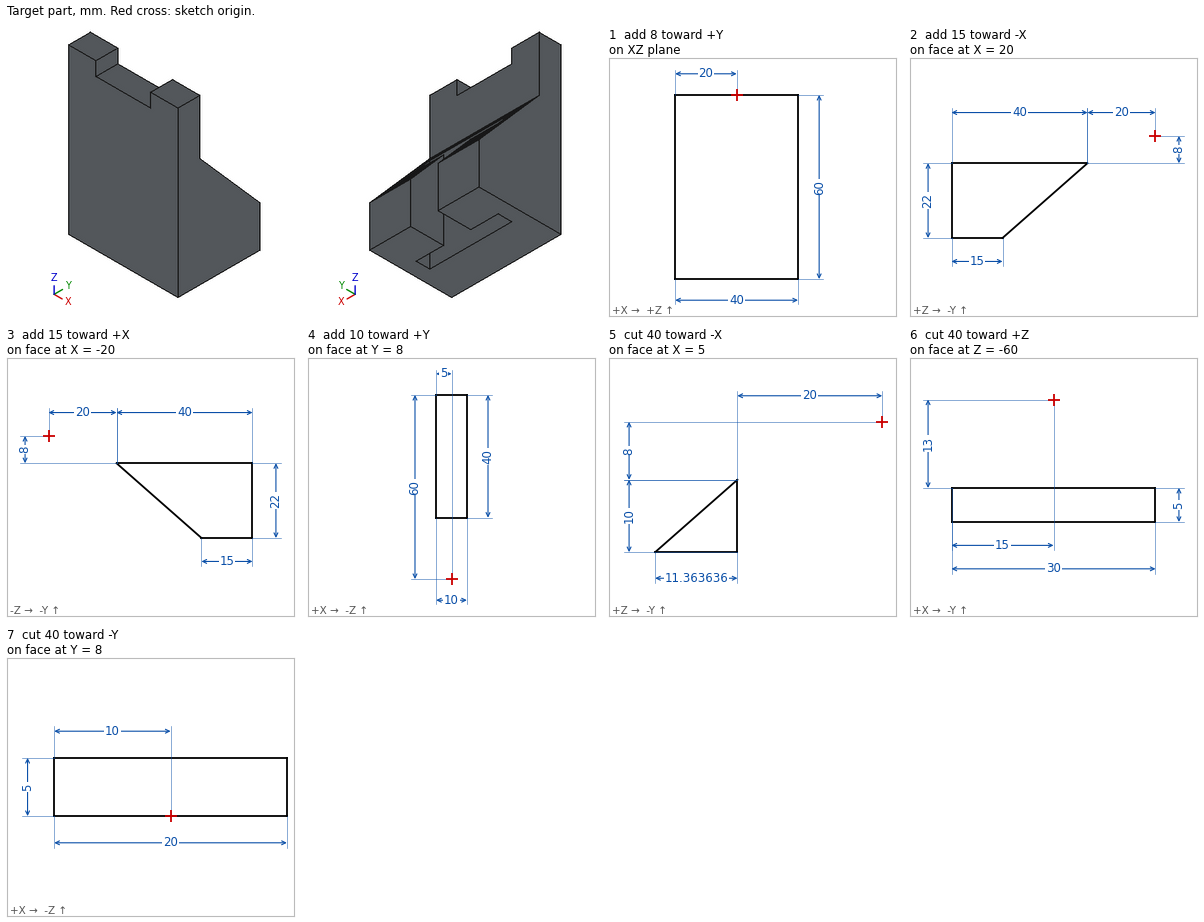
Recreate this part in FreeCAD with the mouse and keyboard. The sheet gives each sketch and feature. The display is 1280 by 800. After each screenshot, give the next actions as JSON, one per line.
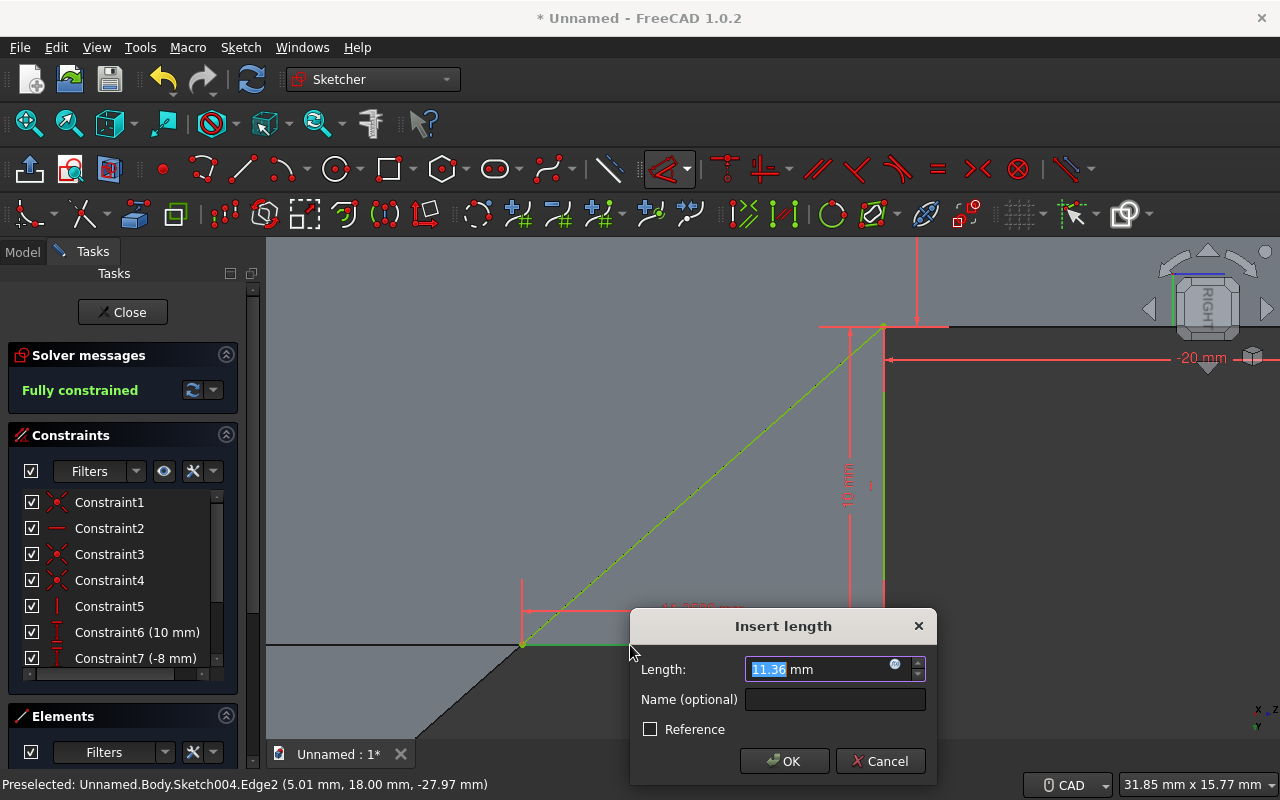
{"action": "type", "text": "11.363636"}
{"action": "key", "text": "Return"}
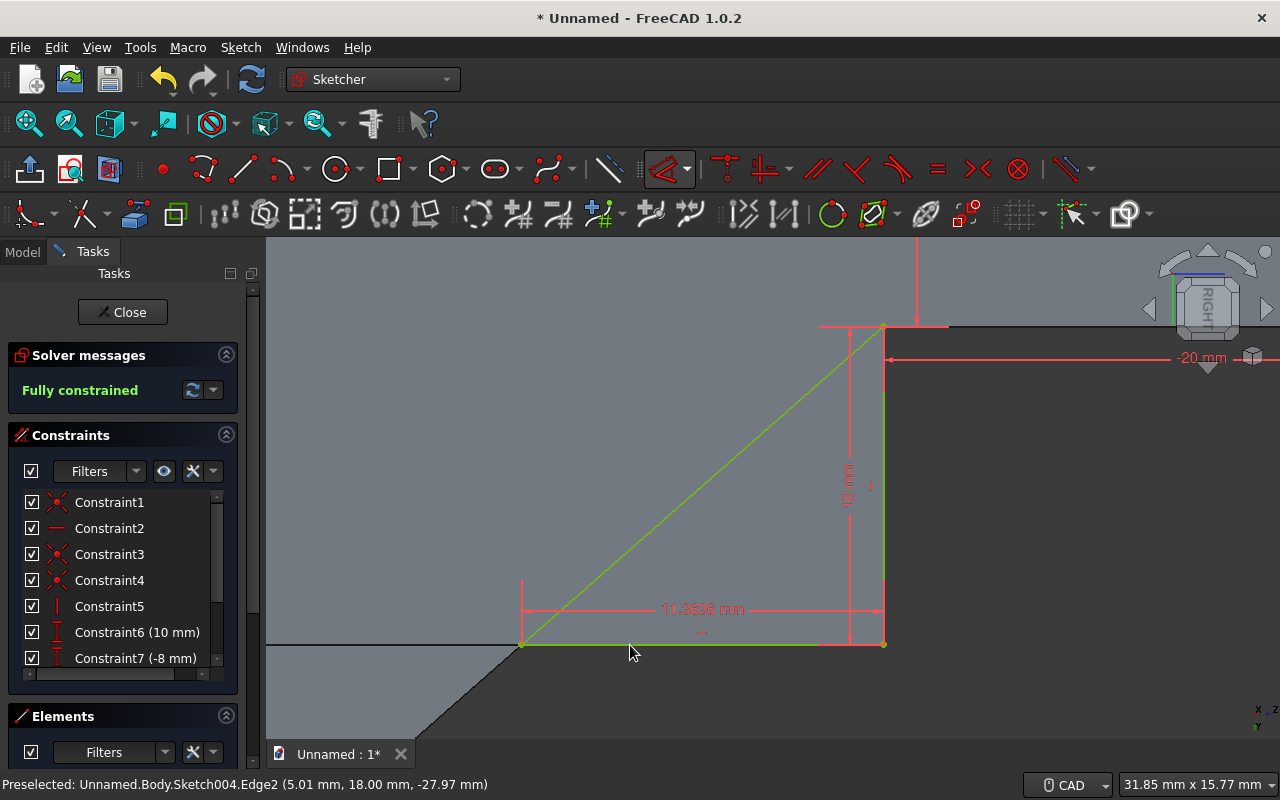
{"action": "left_click", "coordinate": [123, 312]}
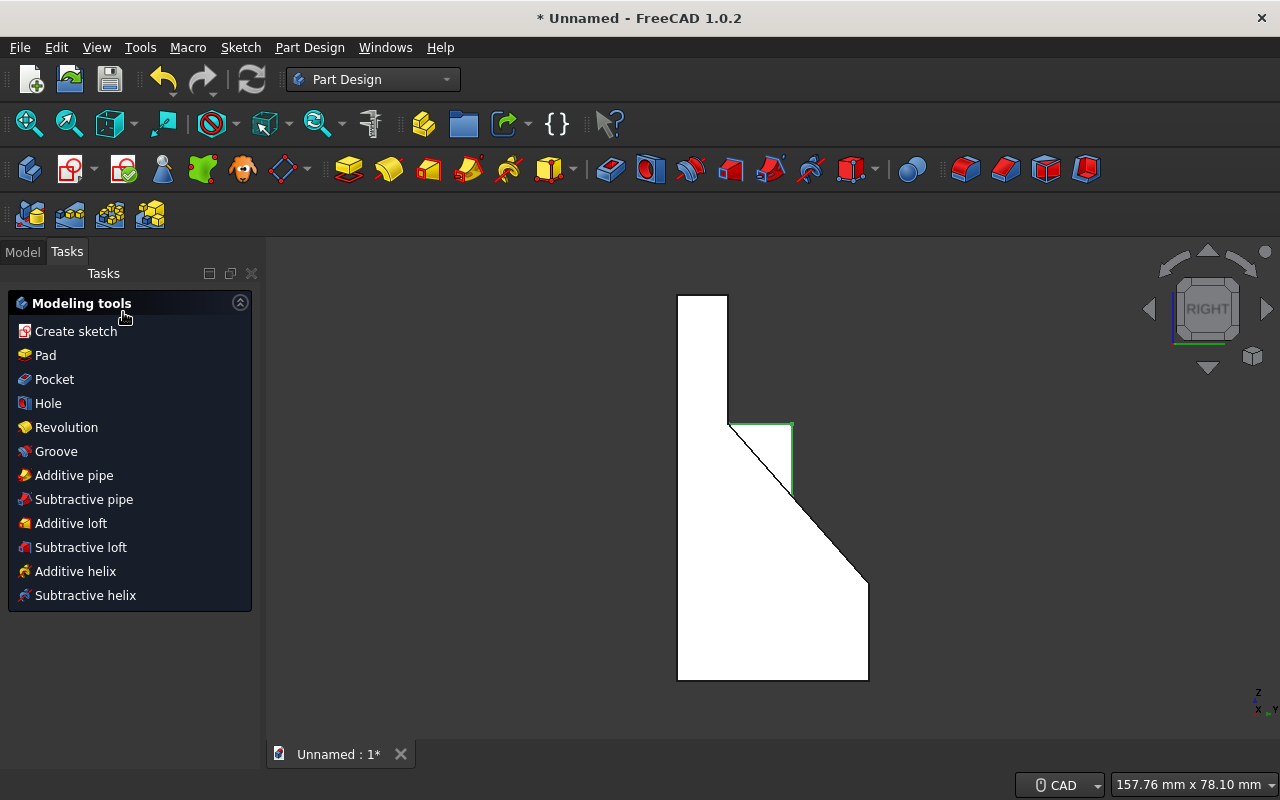
{"action": "left_click", "coordinate": [612, 170]}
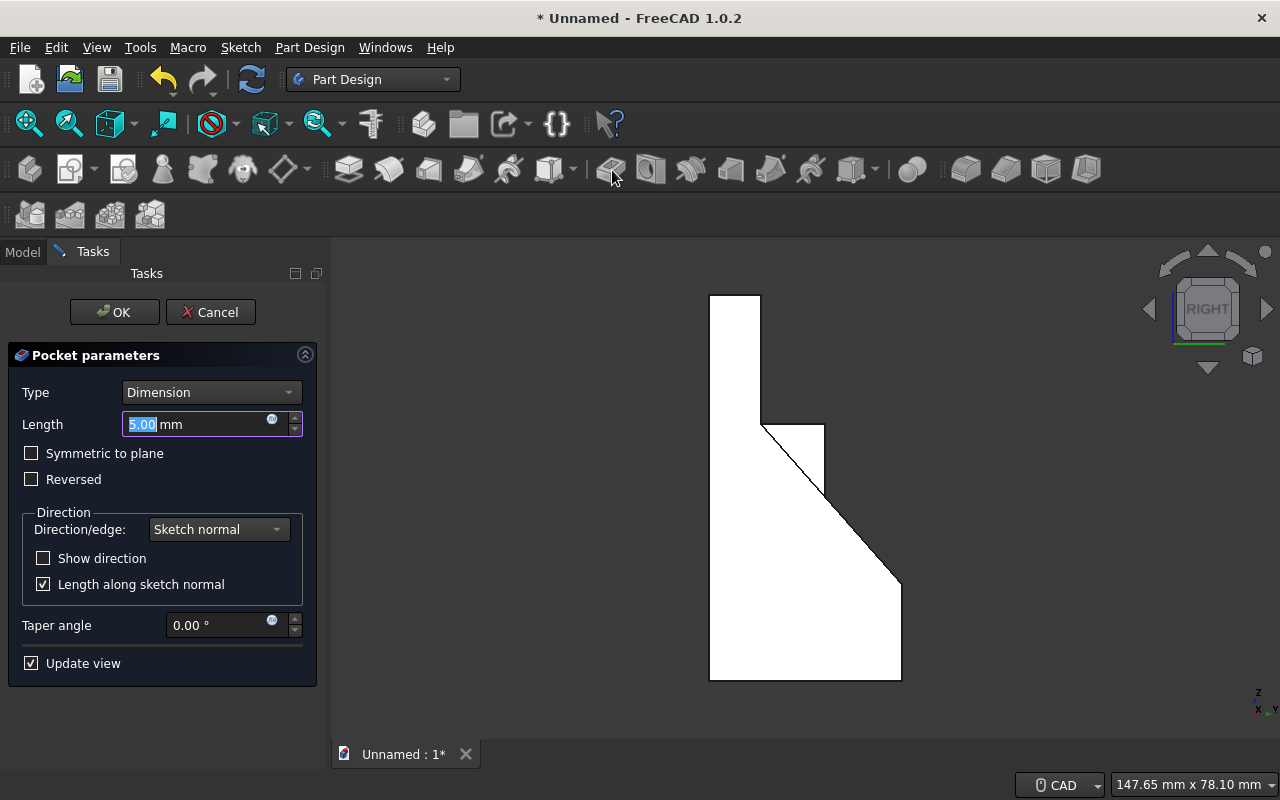
{"action": "type", "text": "40"}
{"action": "key", "text": "Tab"}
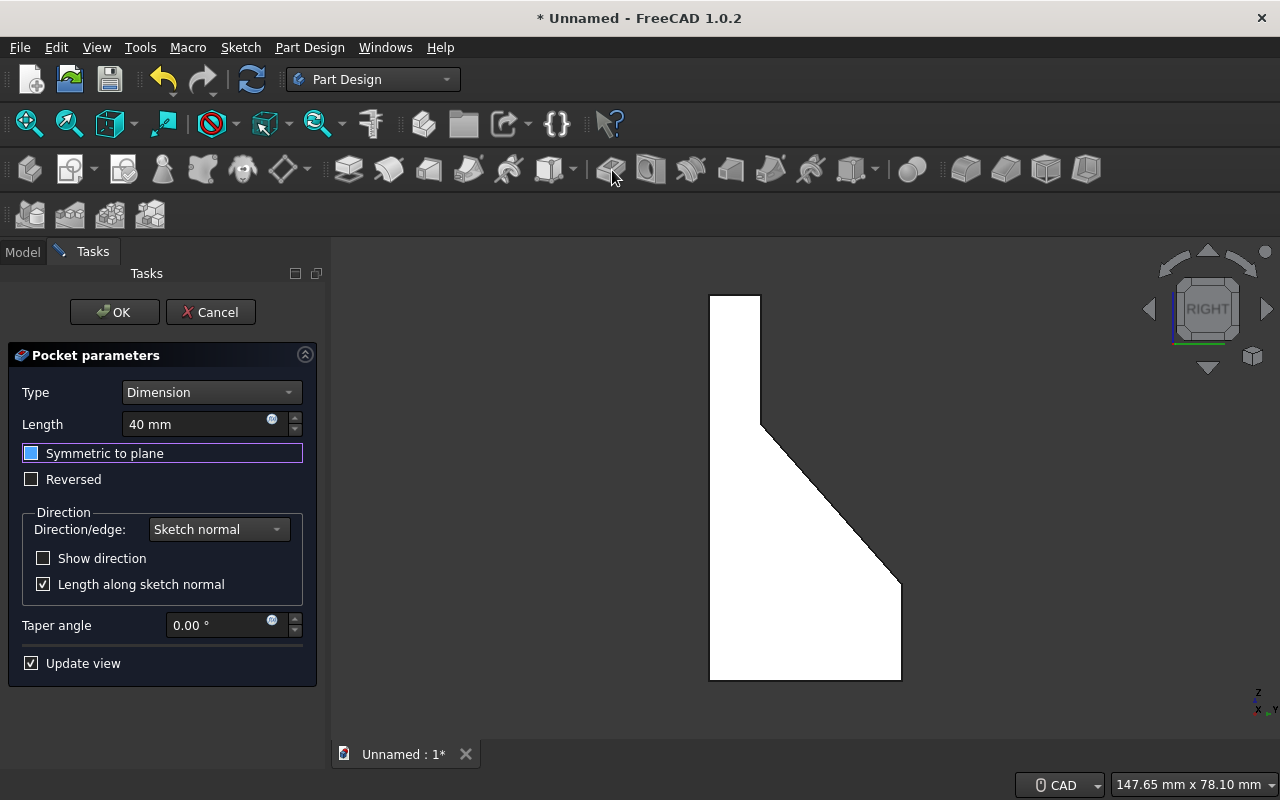
{"action": "left_click", "coordinate": [115, 312]}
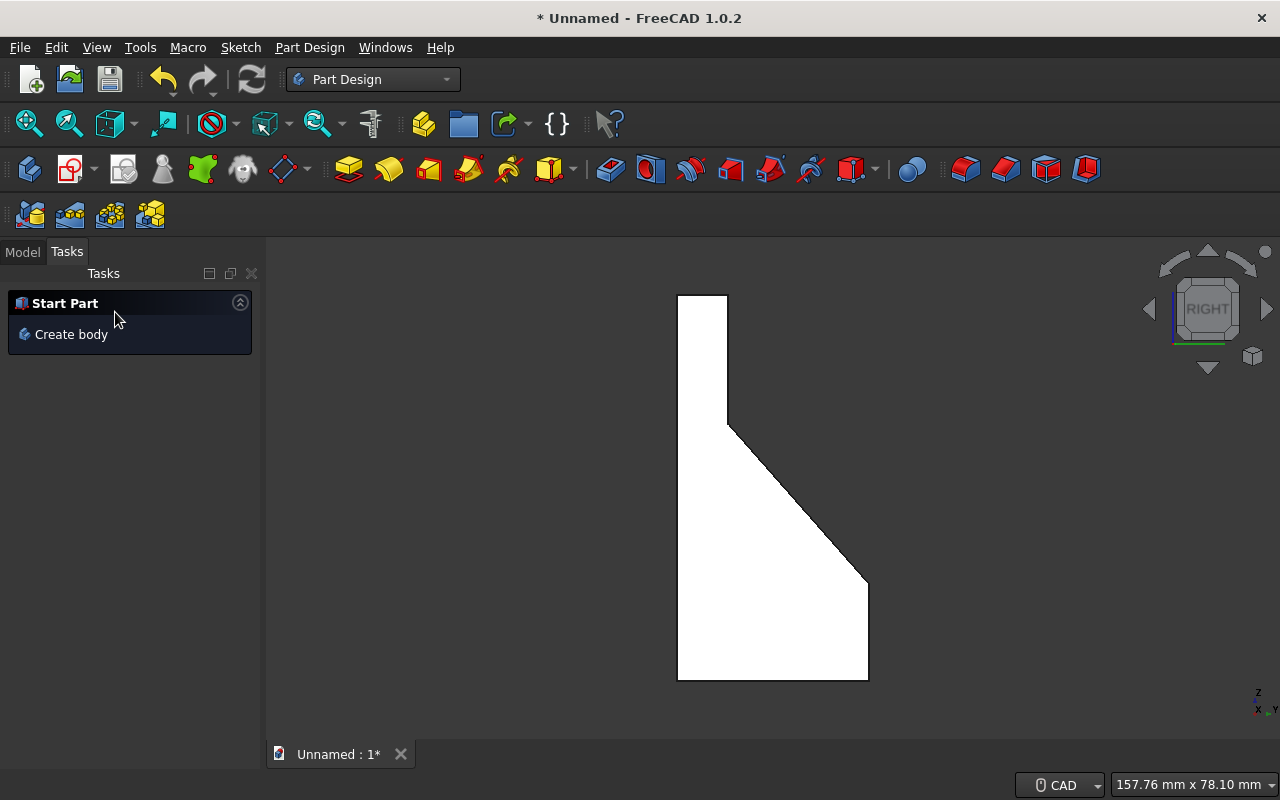
{"action": "key", "text": "5"}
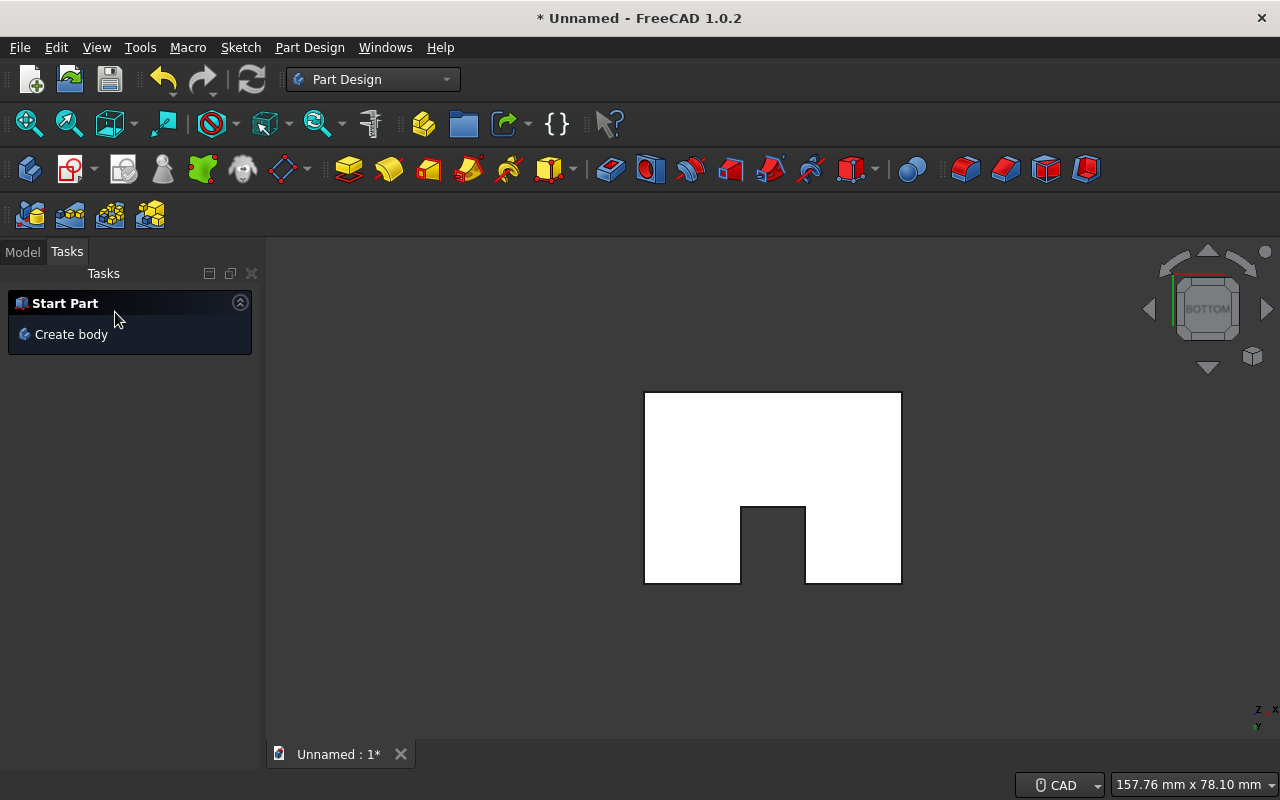
{"action": "left_click", "coordinate": [30, 124]}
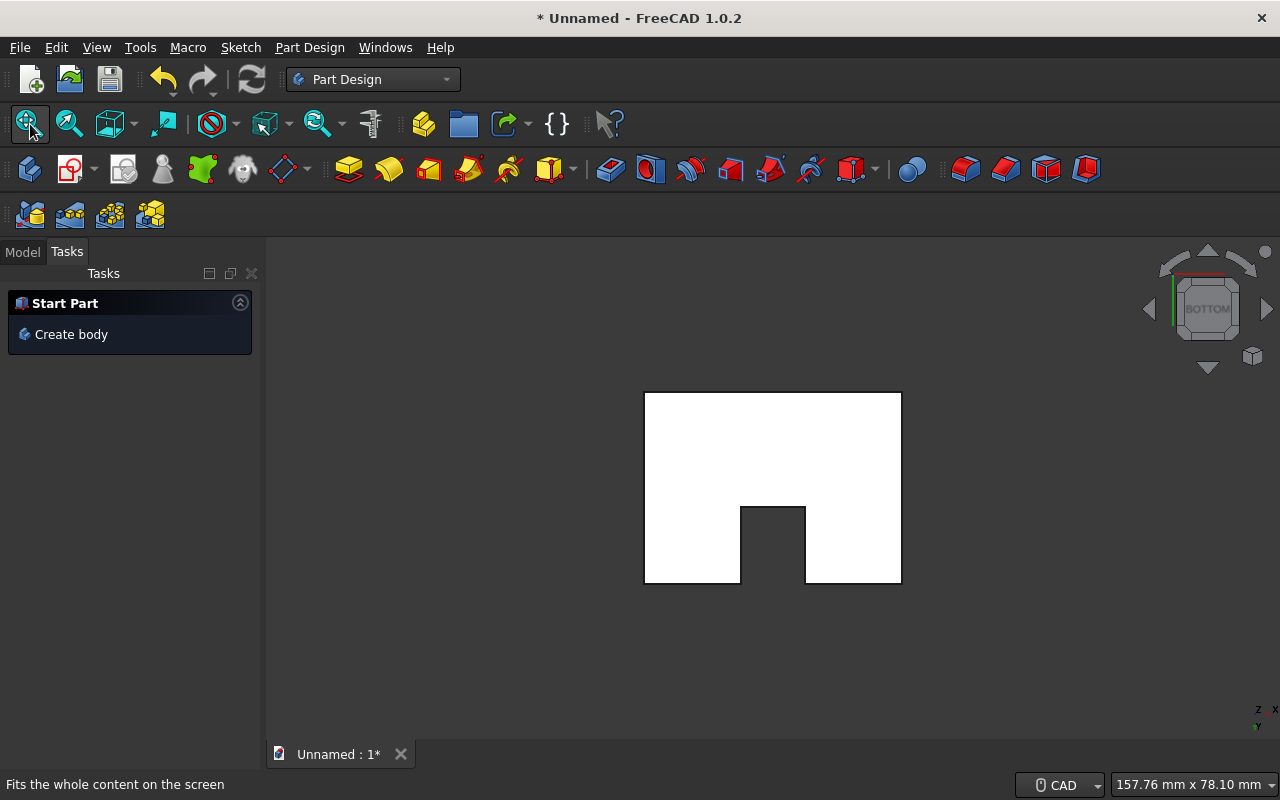
{"action": "left_click", "coordinate": [846, 459]}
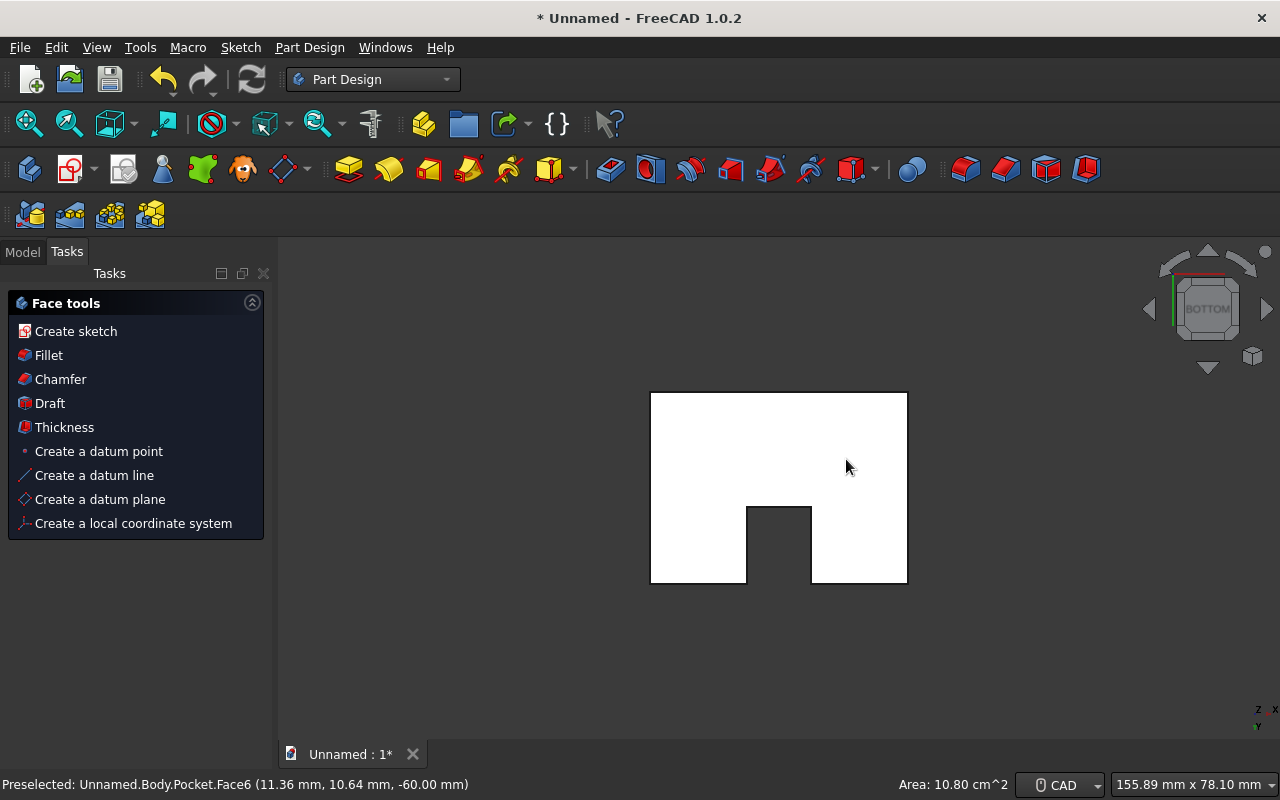
{"action": "left_click", "coordinate": [70, 170]}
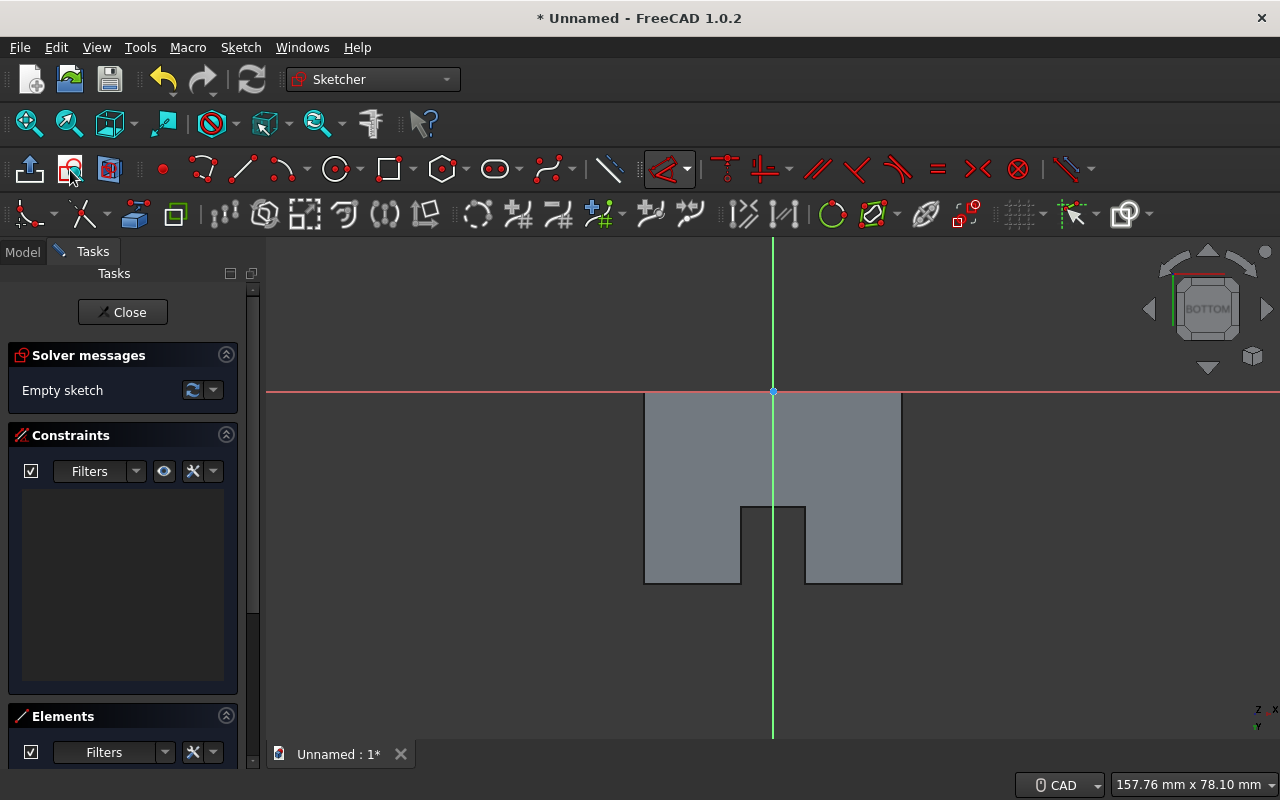
{"action": "scroll", "coordinate": [813, 427], "scroll_direction": "up", "scroll_amount": 5}